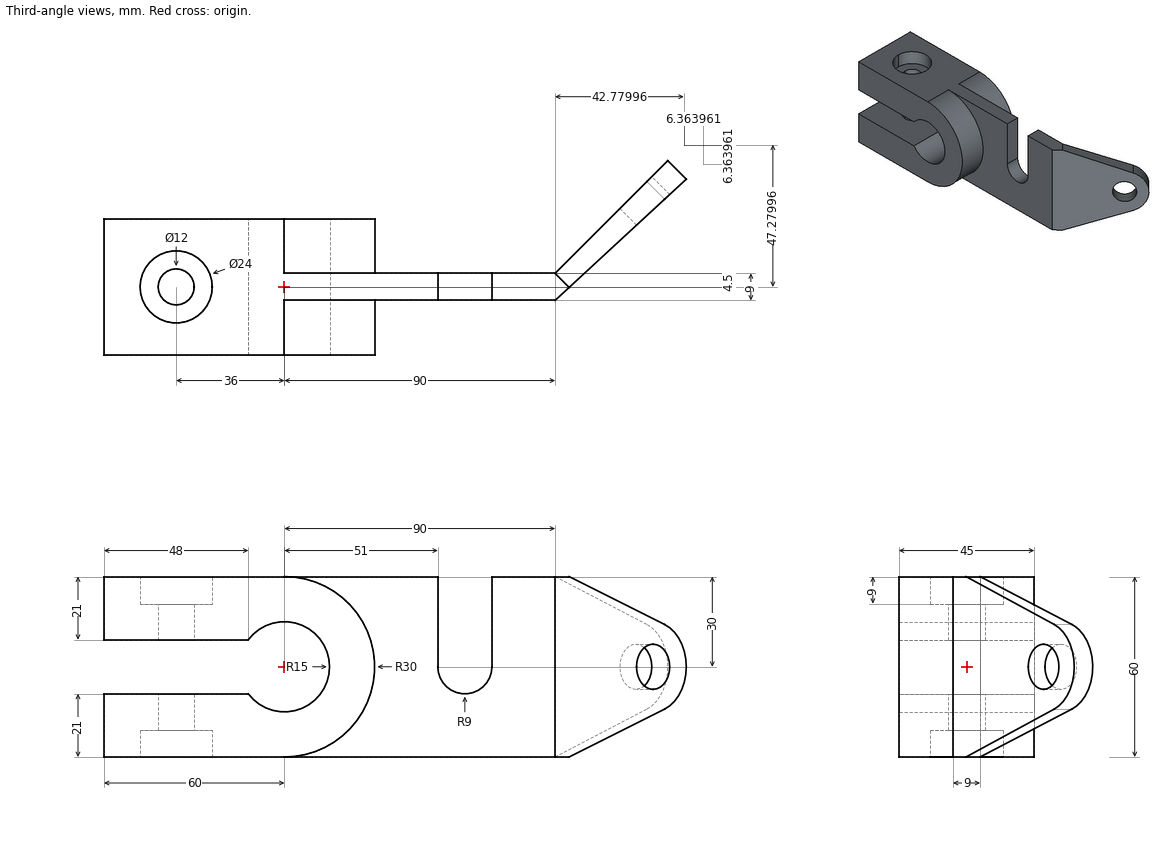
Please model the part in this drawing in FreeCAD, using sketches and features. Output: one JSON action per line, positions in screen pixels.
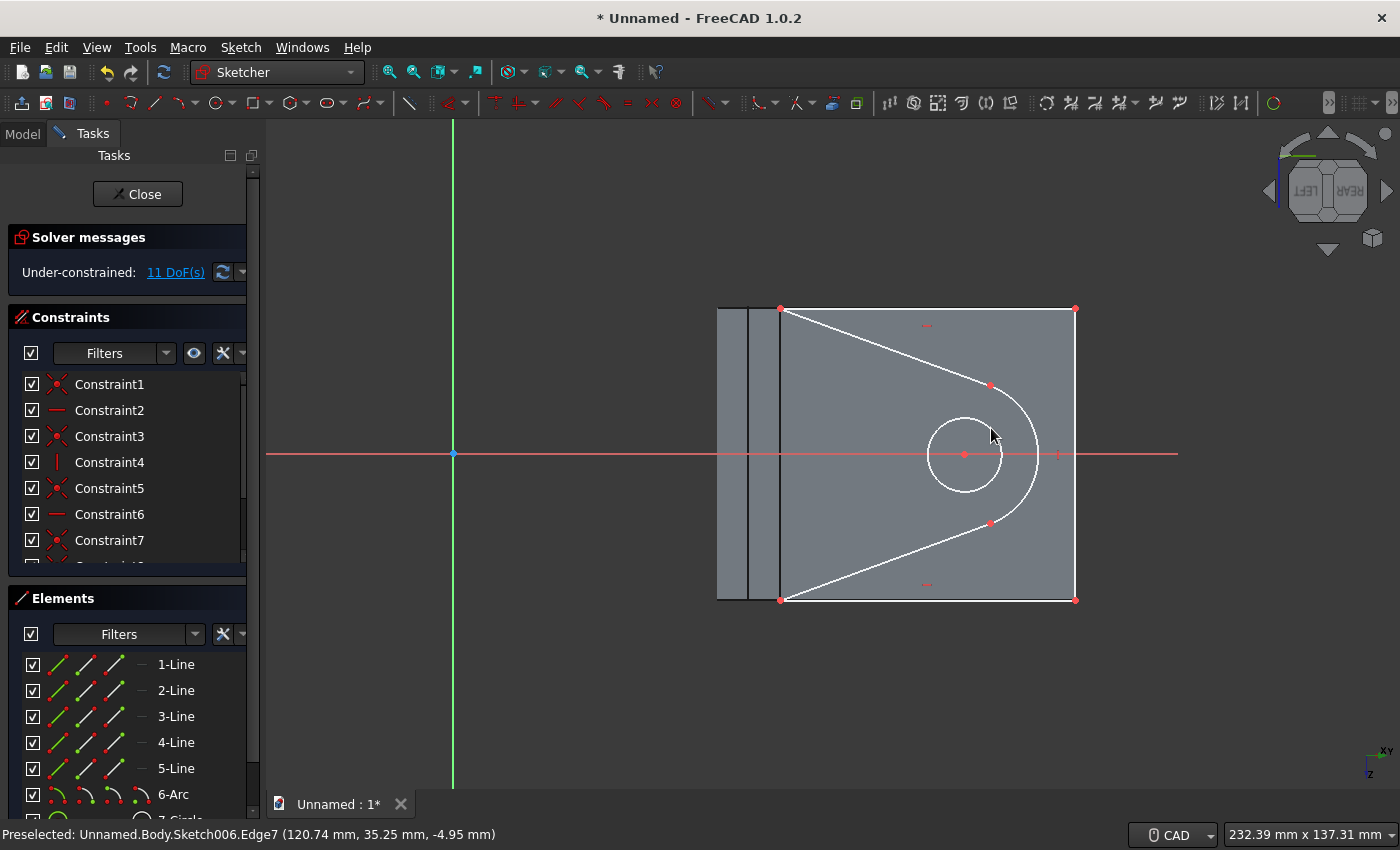
{"action": "left_click", "coordinate": [927, 547]}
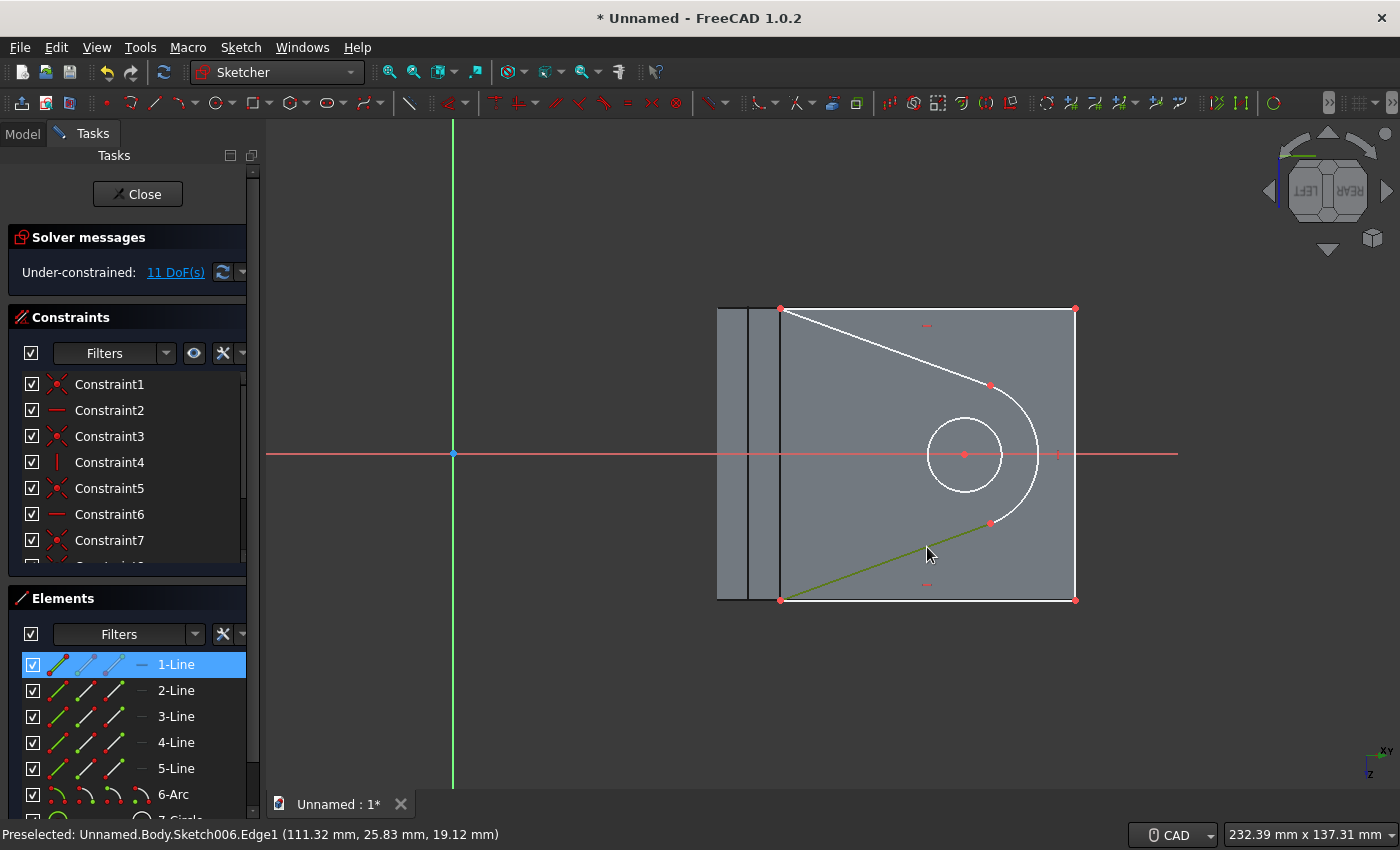
{"action": "left_click", "coordinate": [1030, 489]}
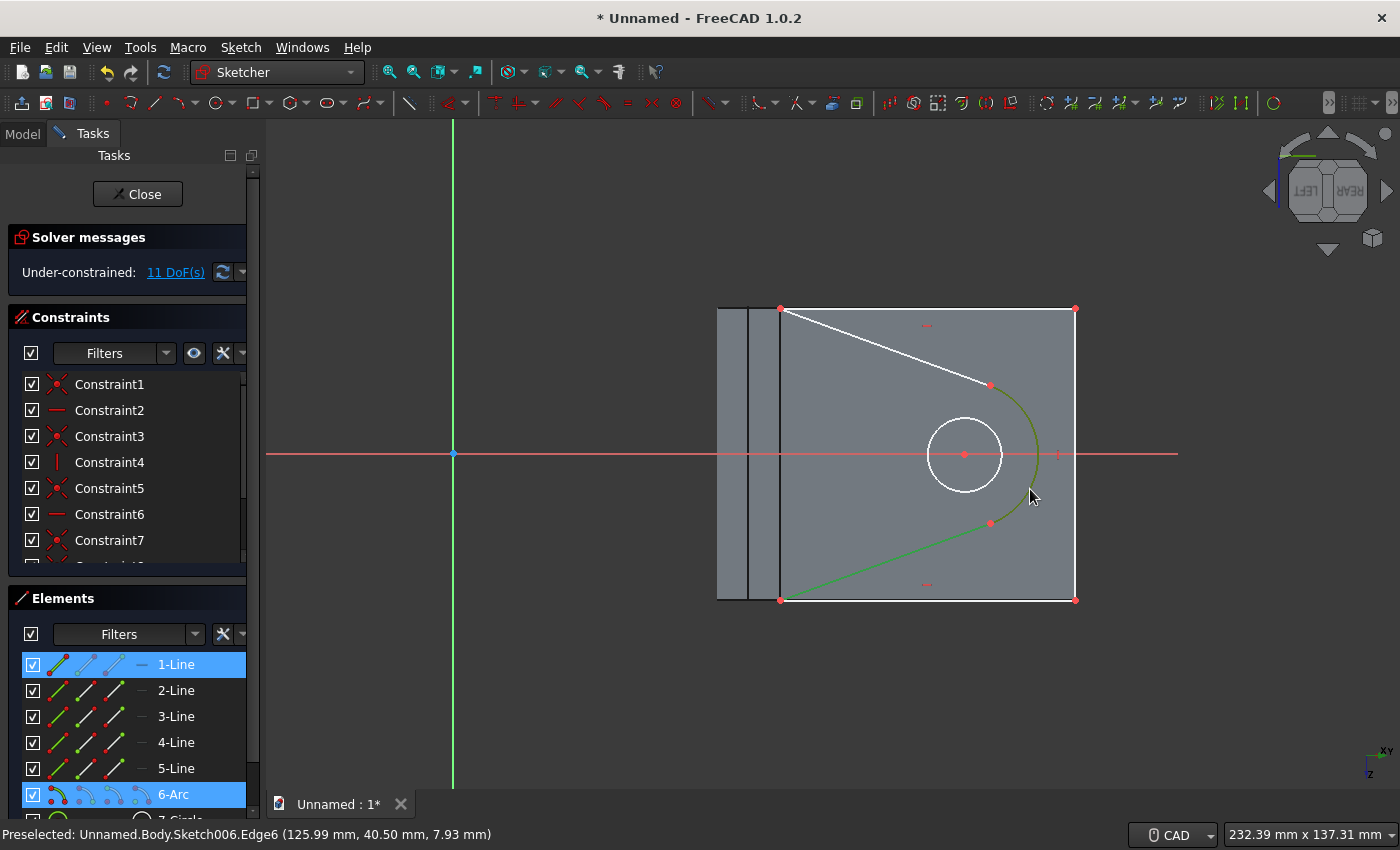
{"action": "left_click", "coordinate": [604, 104]}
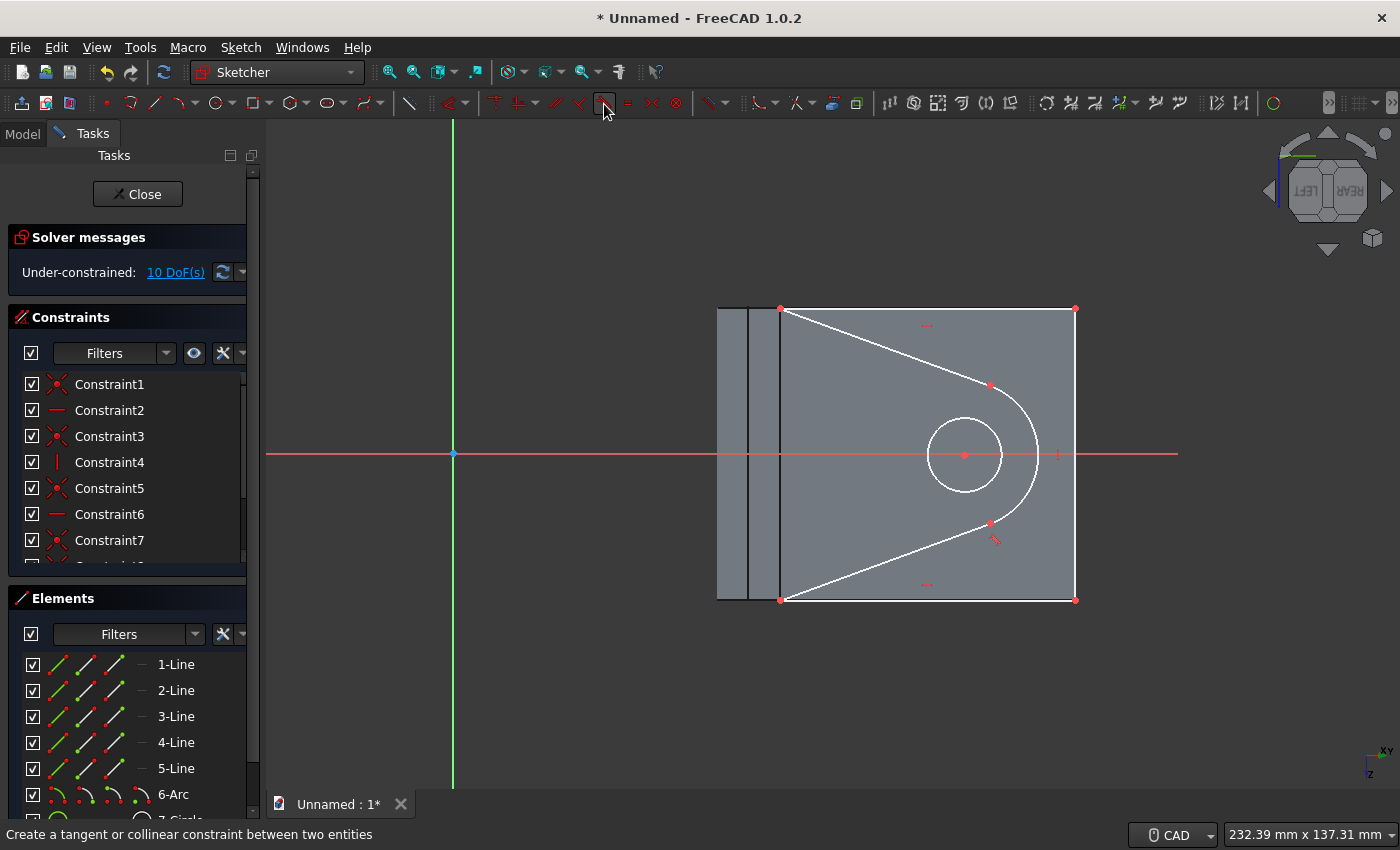
{"action": "left_click", "coordinate": [843, 332]}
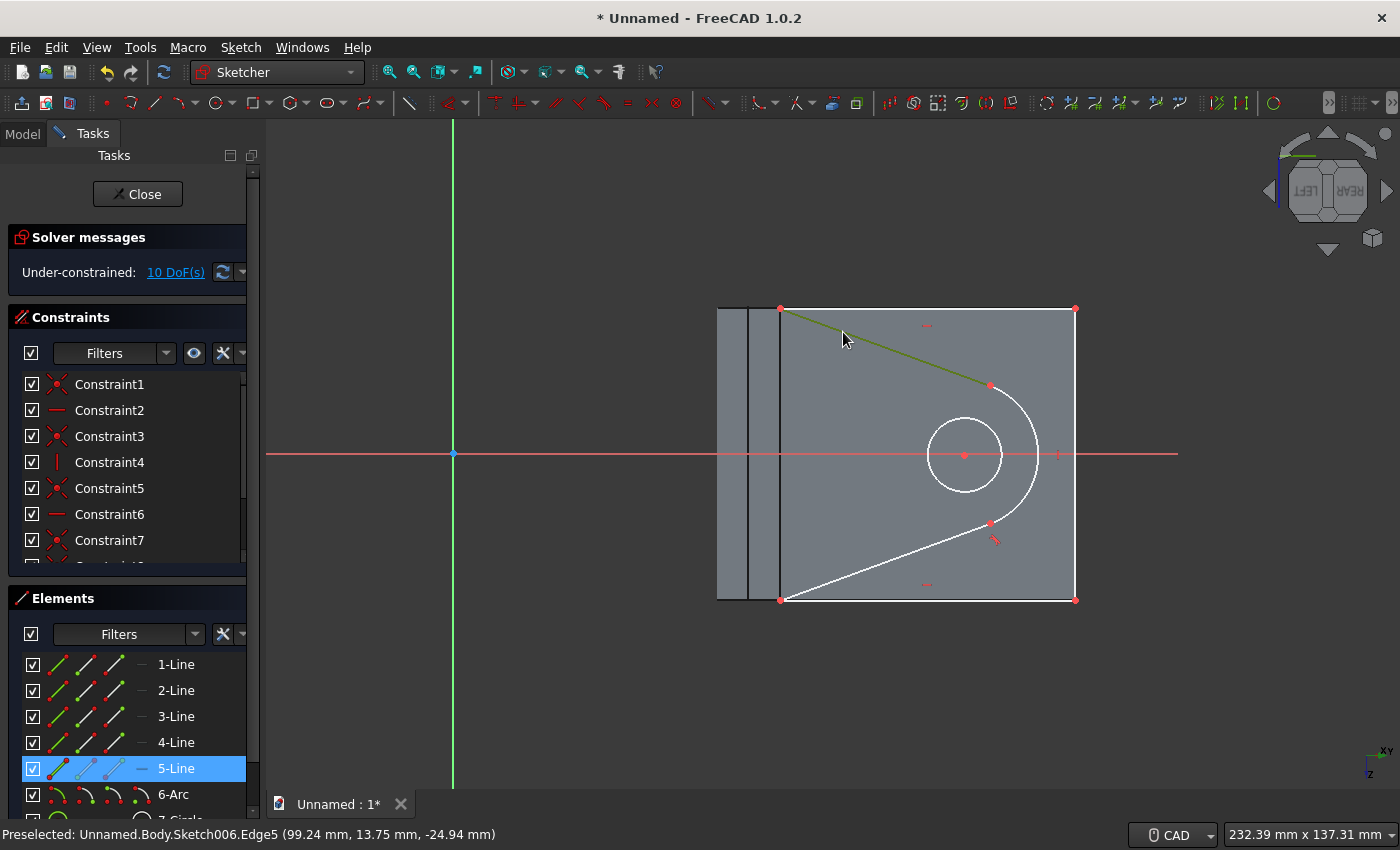
{"action": "left_click", "coordinate": [1030, 489]}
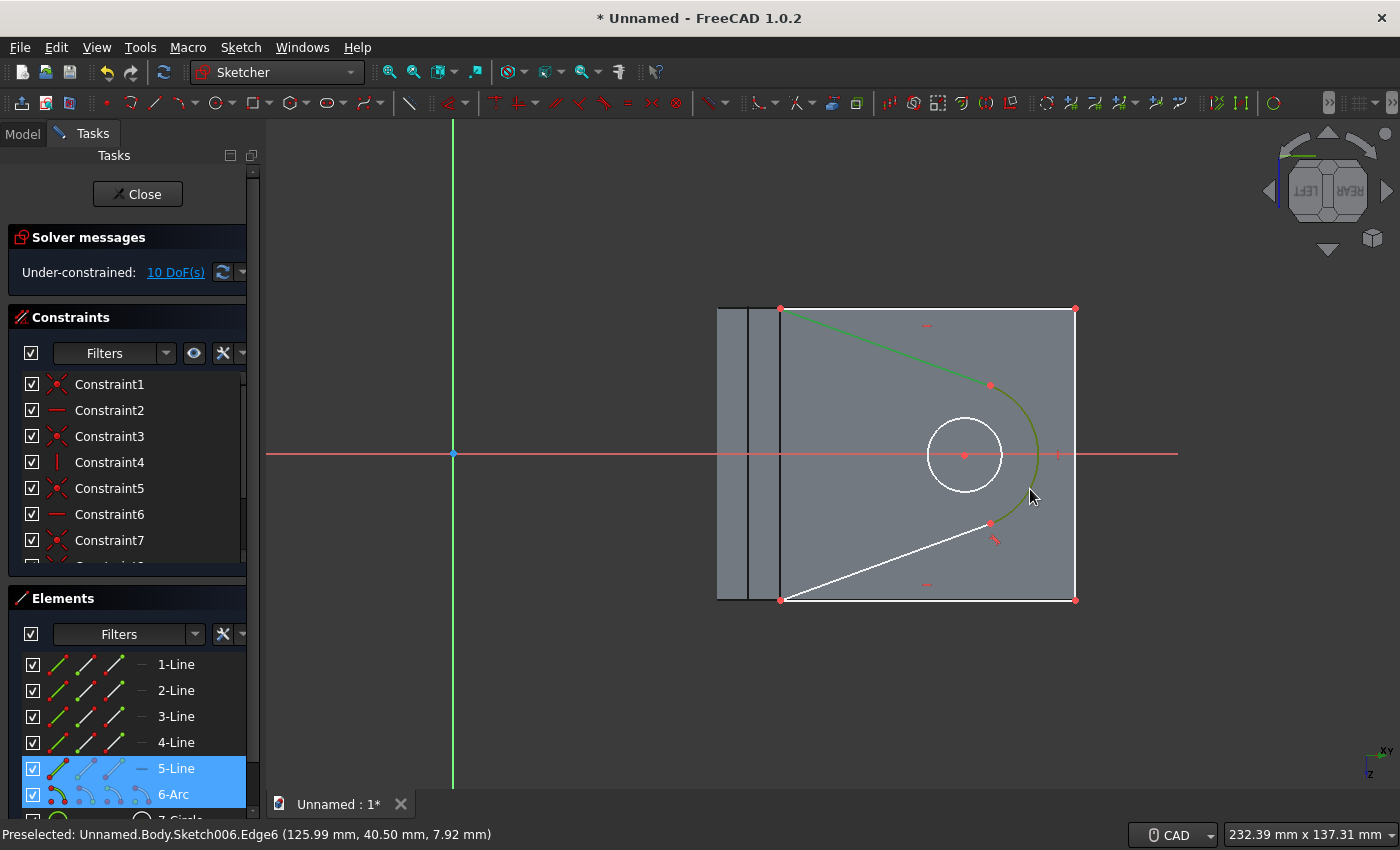
{"action": "key", "text": "t"}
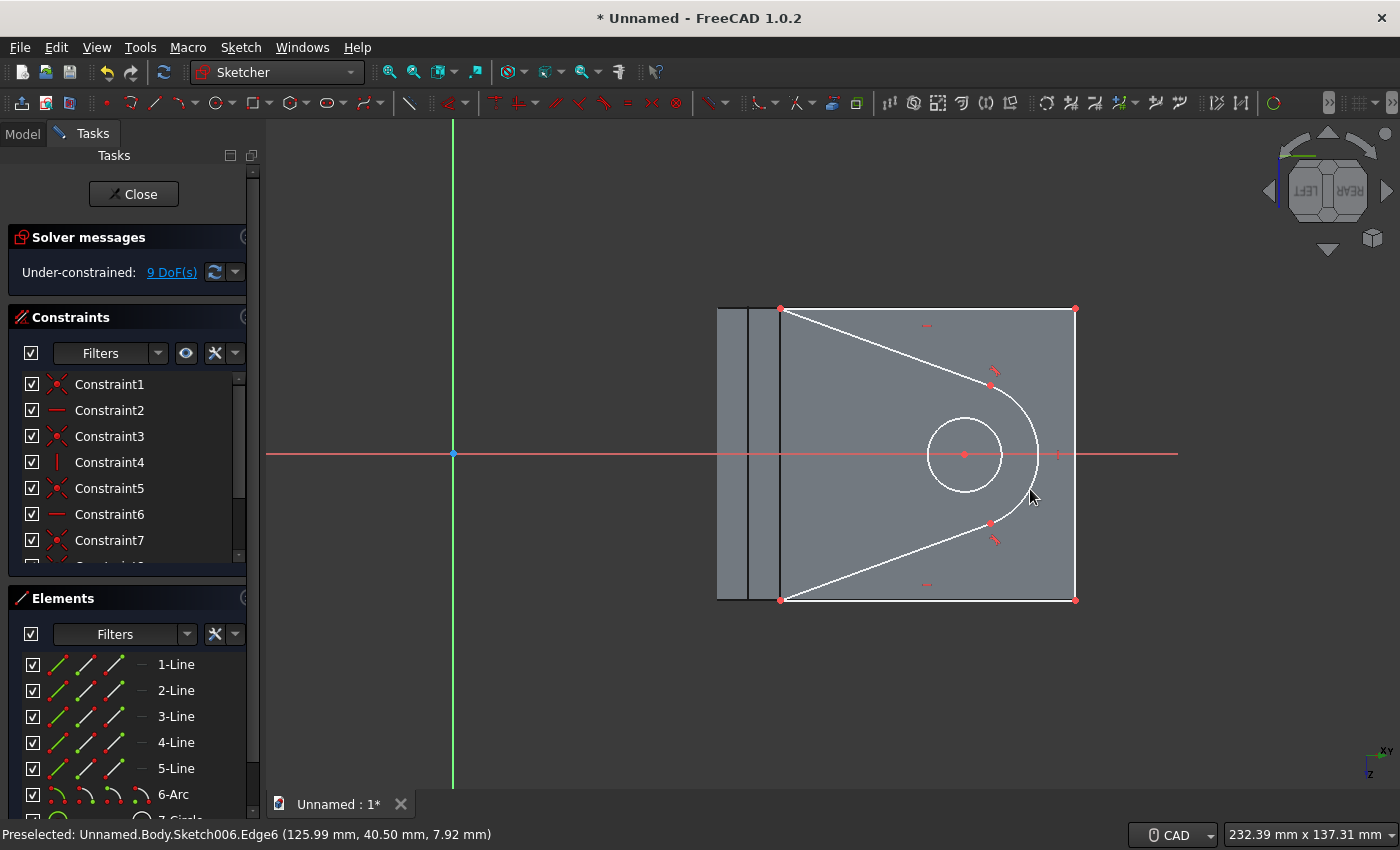
{"action": "left_click", "coordinate": [965, 455]}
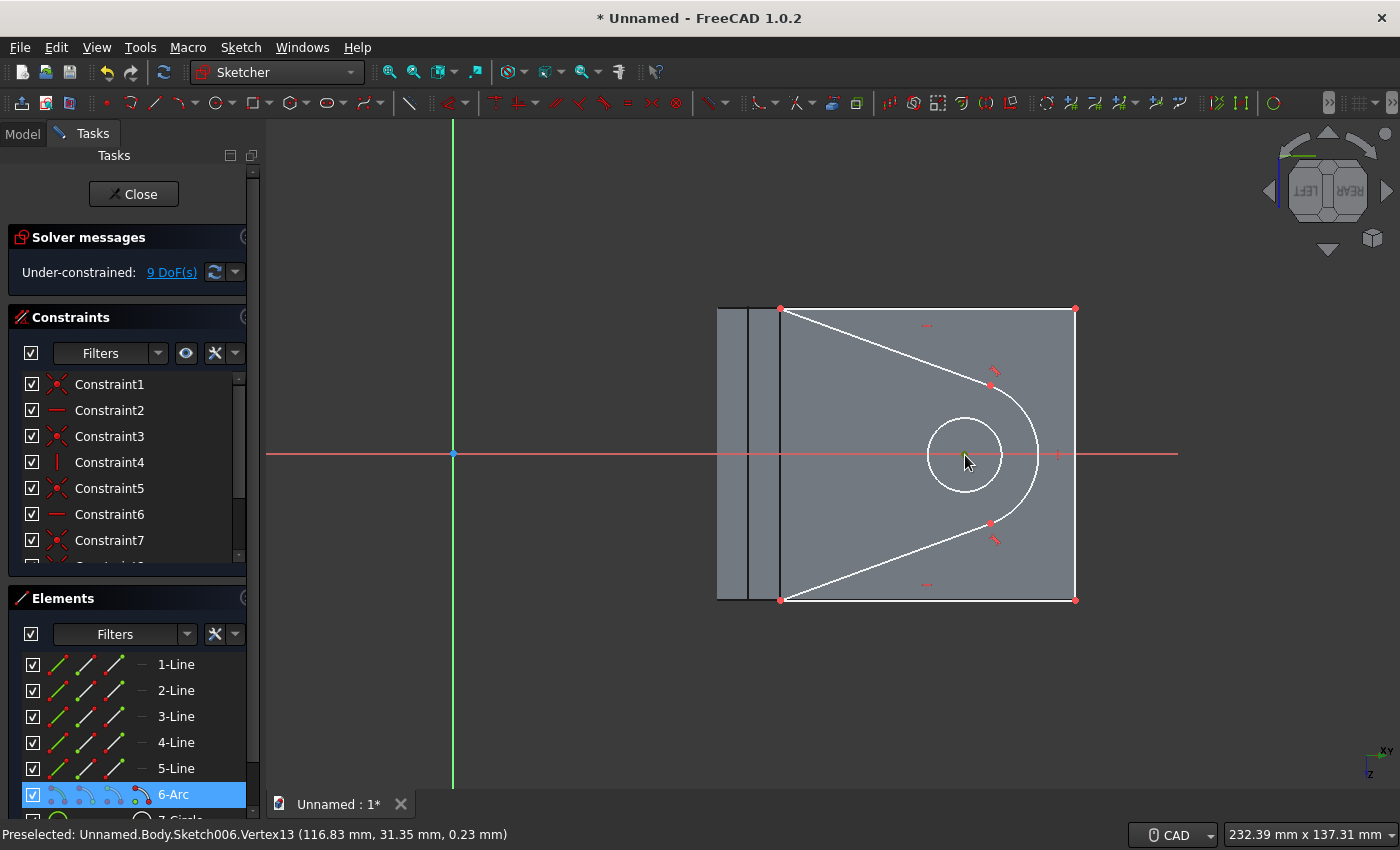
{"action": "left_click", "coordinate": [361, 454]}